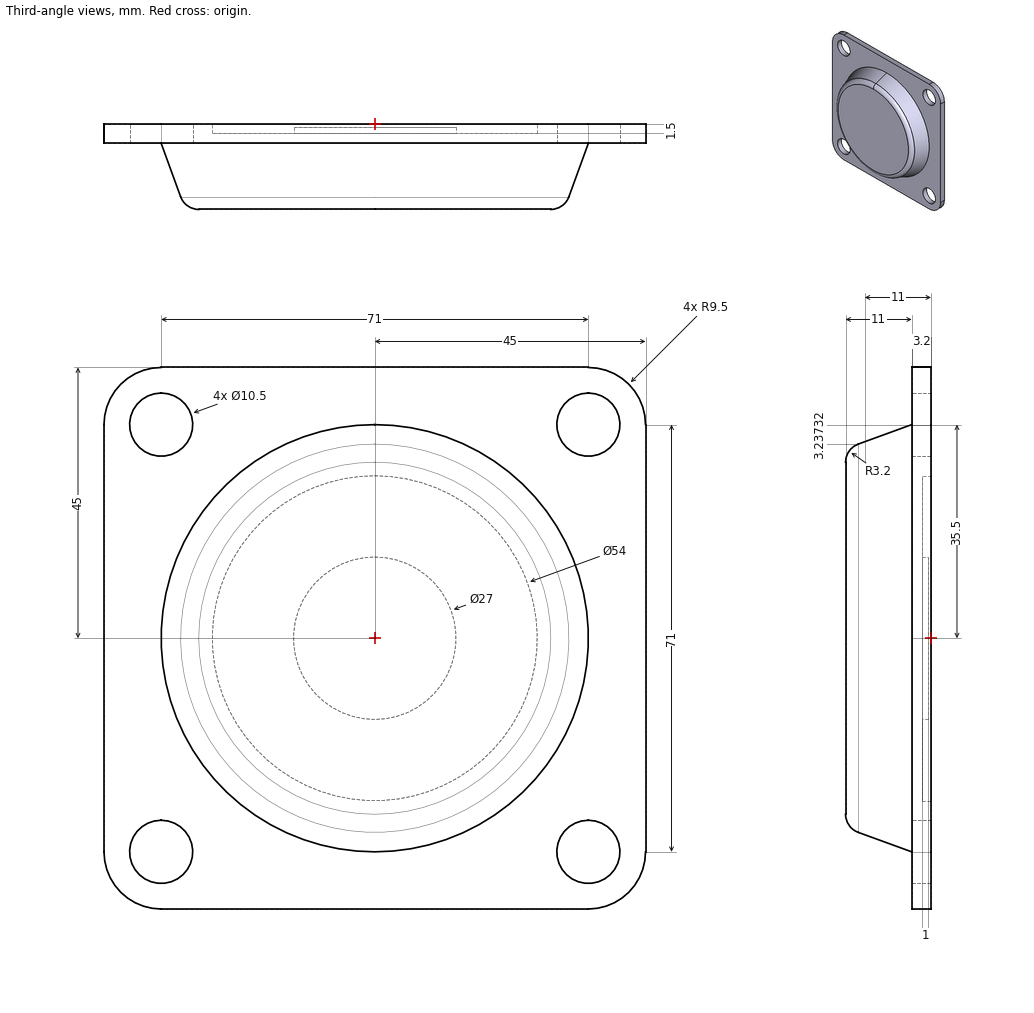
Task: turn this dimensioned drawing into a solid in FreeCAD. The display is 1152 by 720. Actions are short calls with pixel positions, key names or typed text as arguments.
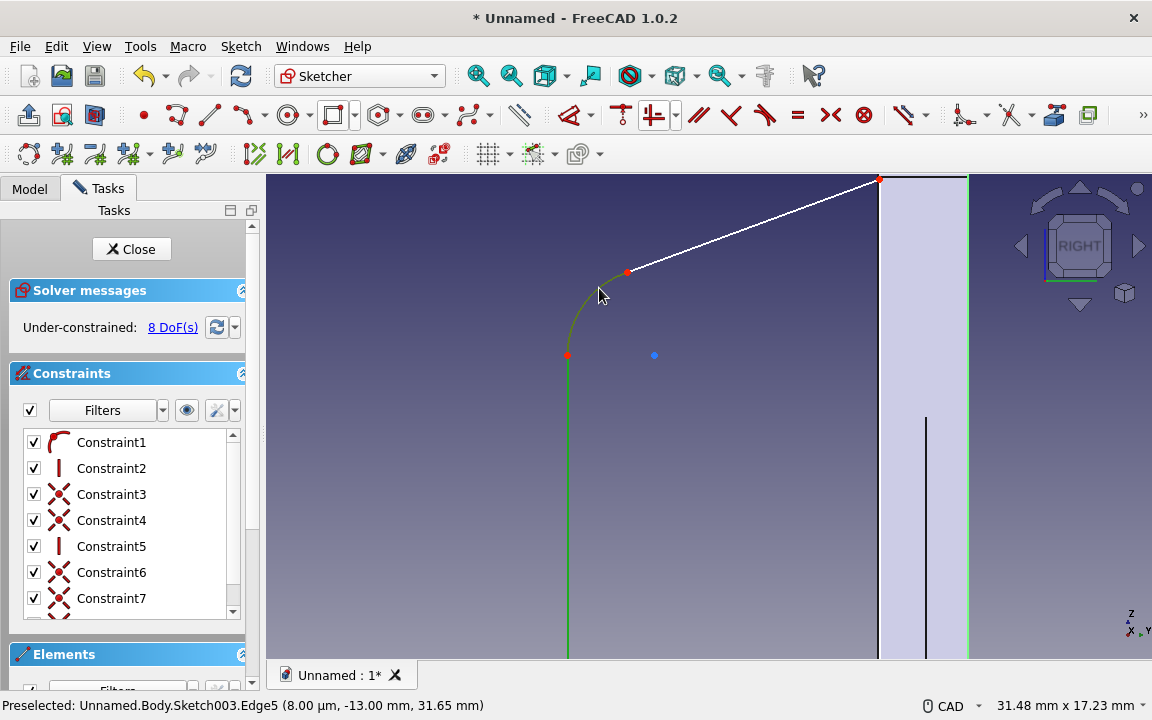
click(765, 116)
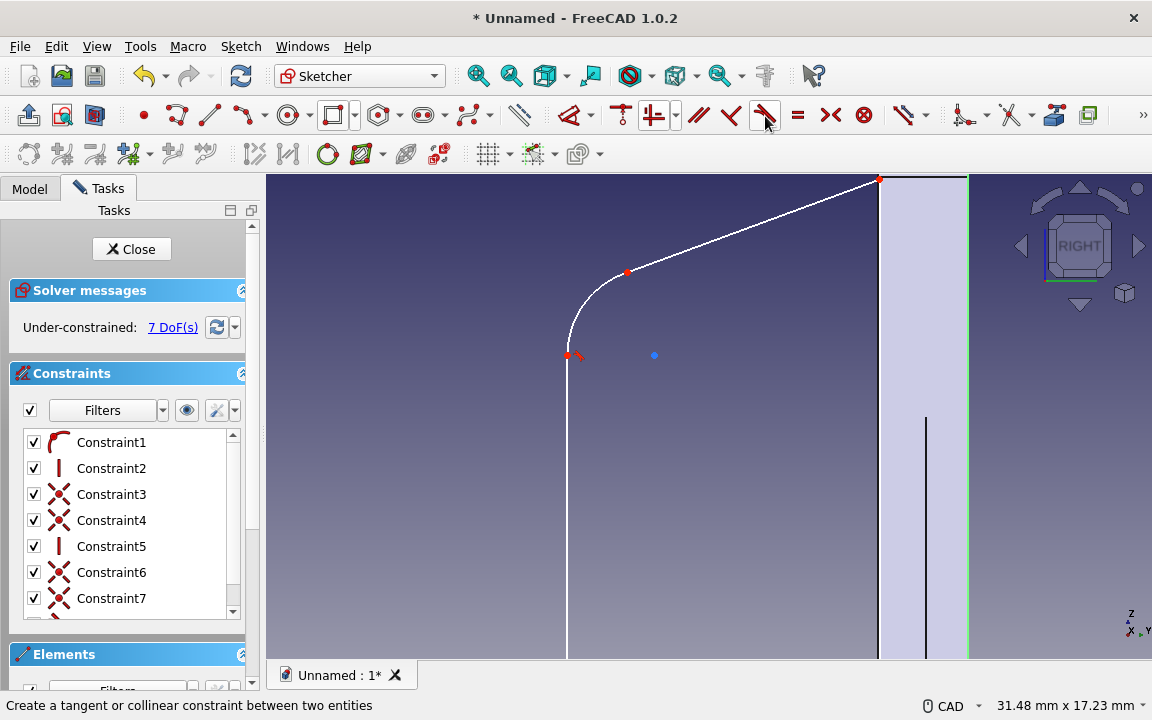
click(804, 207)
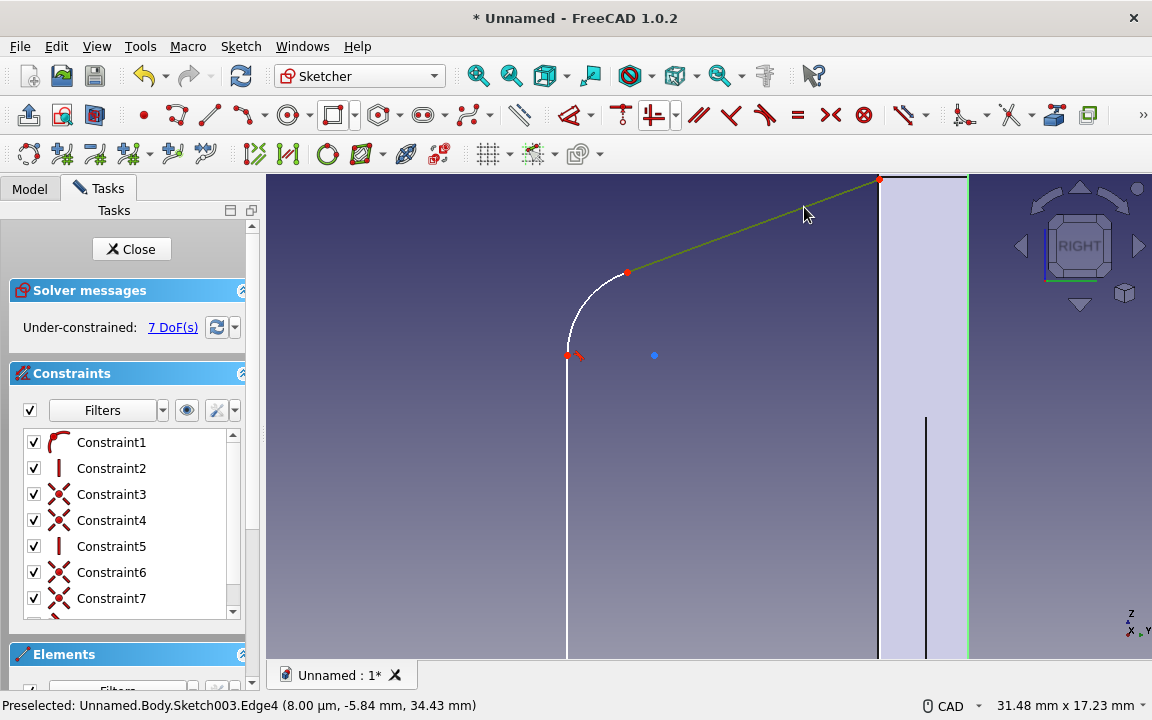
click(599, 288)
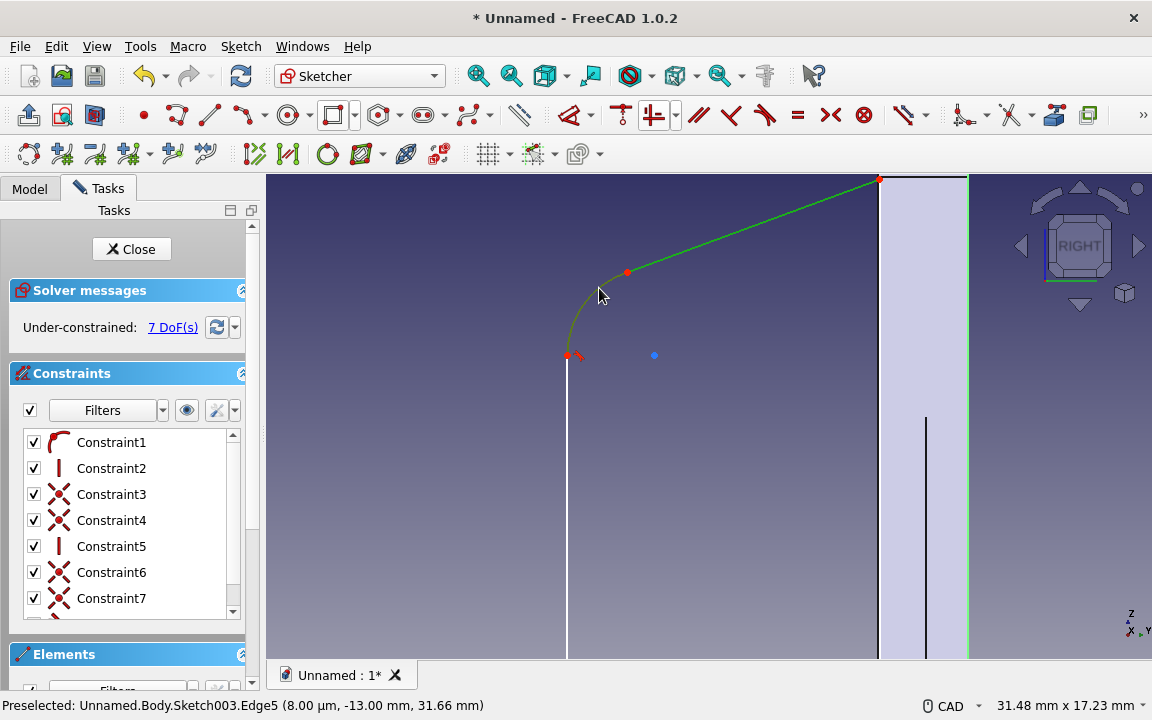
key(t)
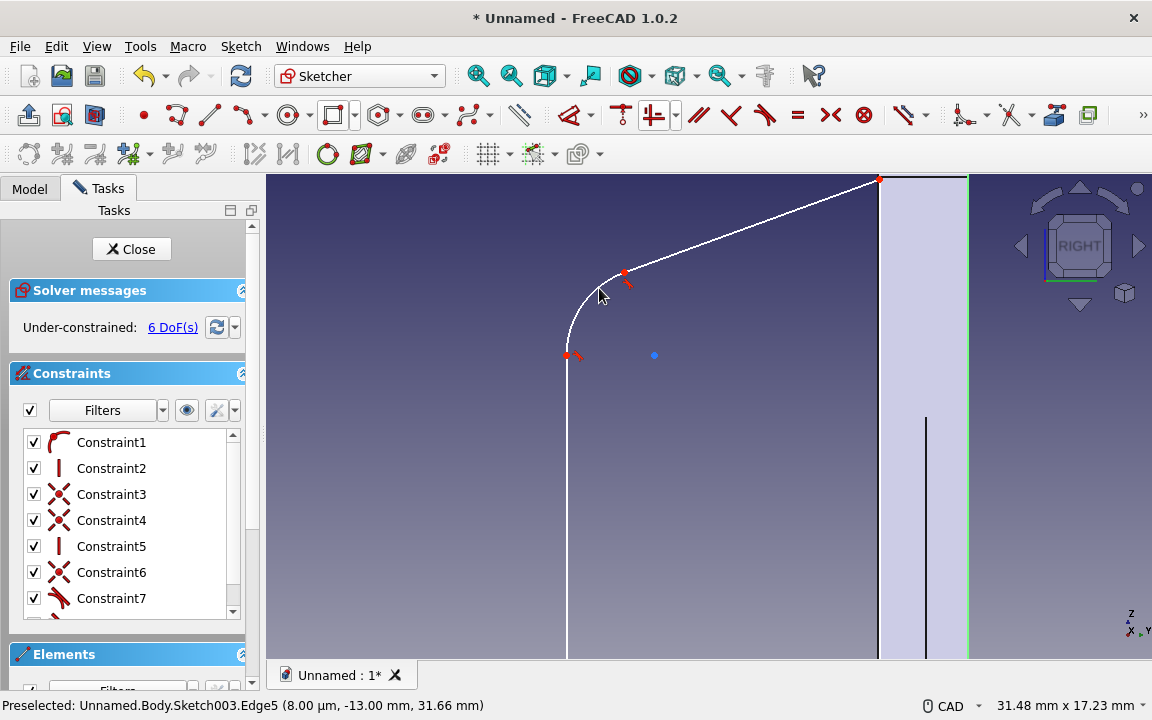
scroll(585, 304, down, 6)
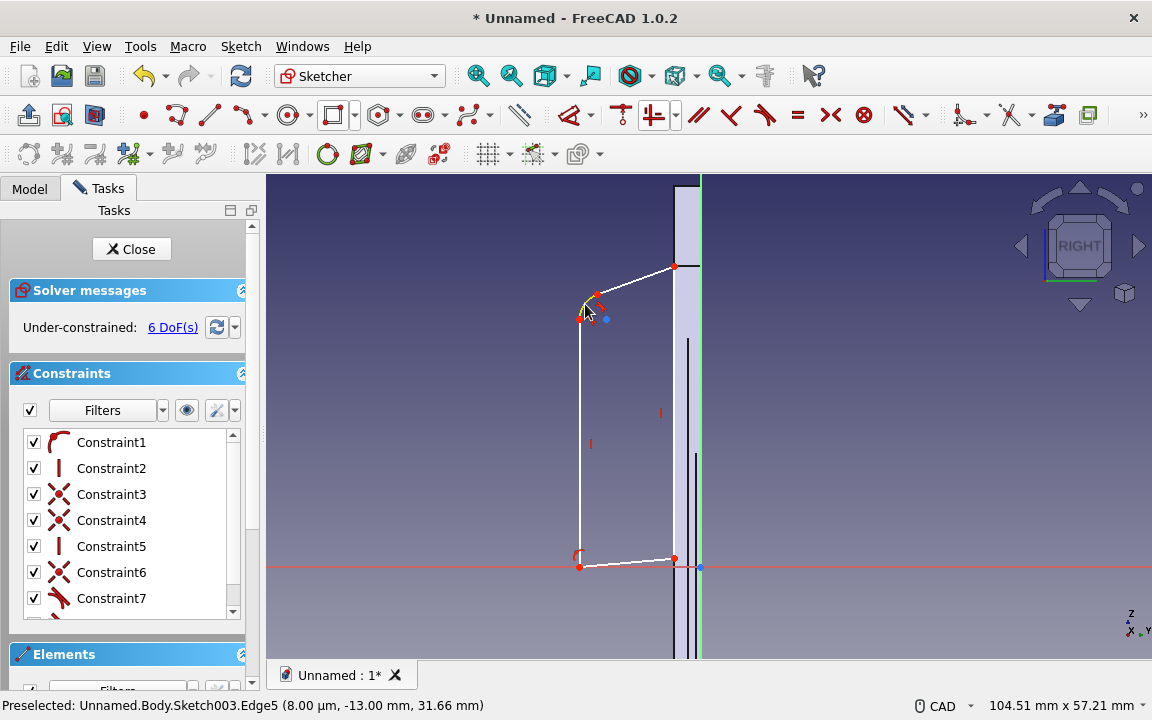
scroll(646, 561, up, 5)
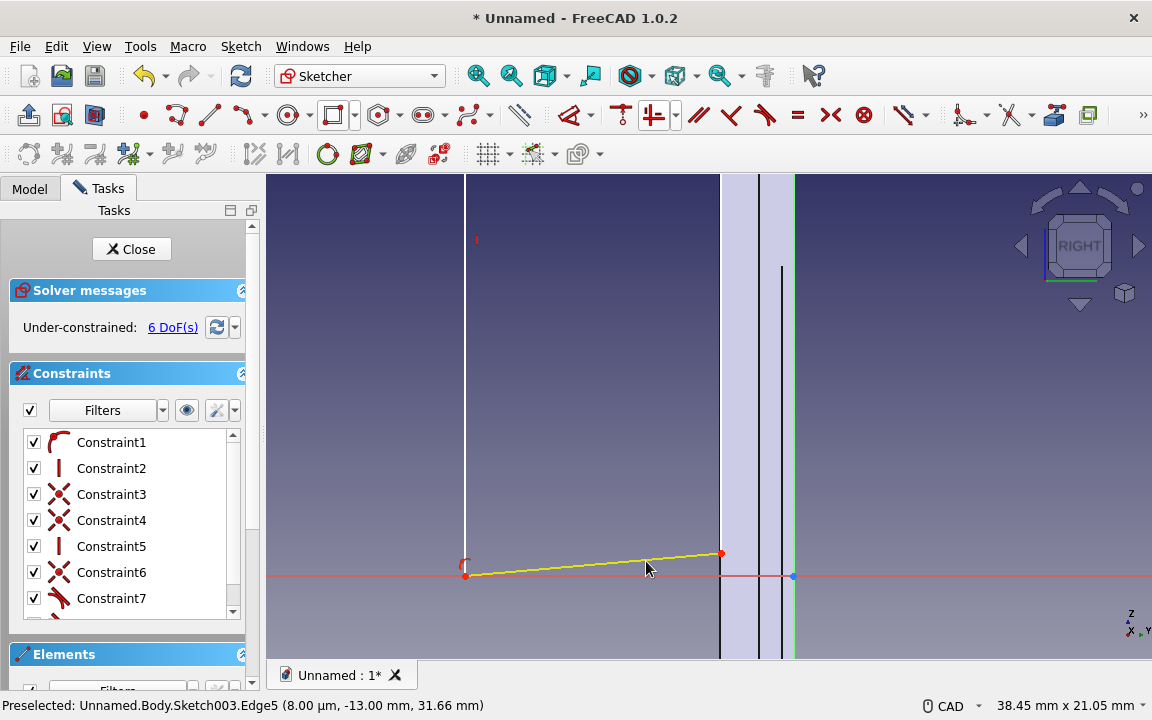
click(644, 560)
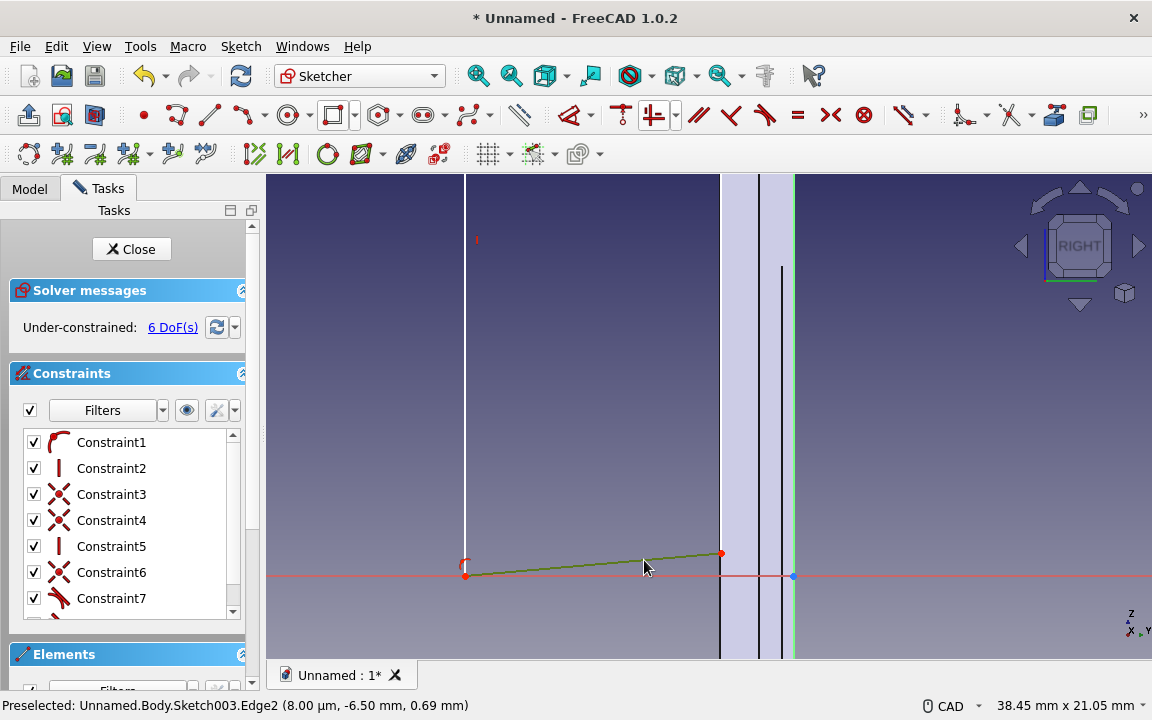
key(h)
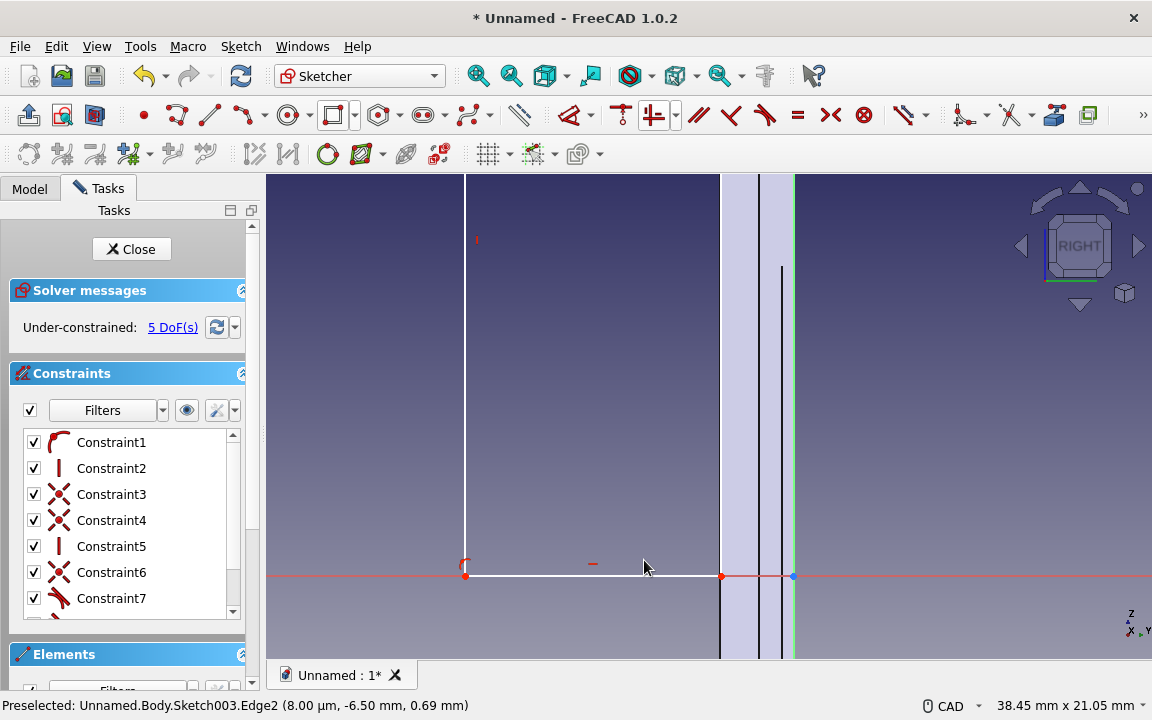
click(568, 116)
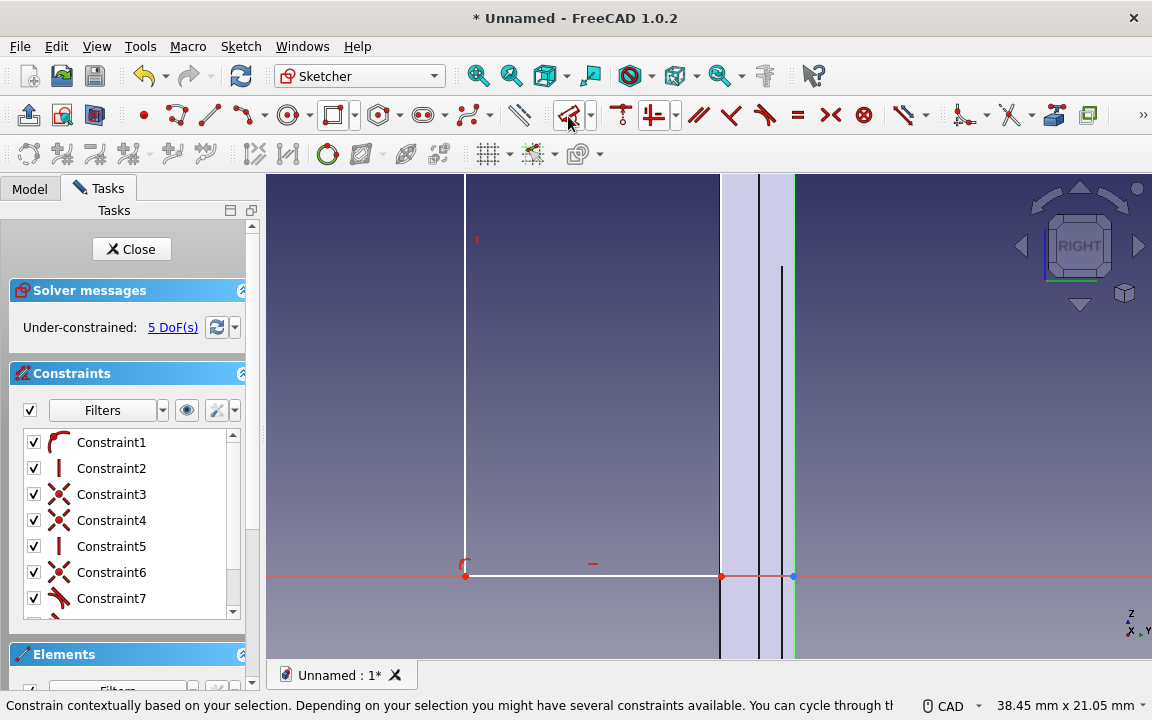
scroll(647, 562, down, 5)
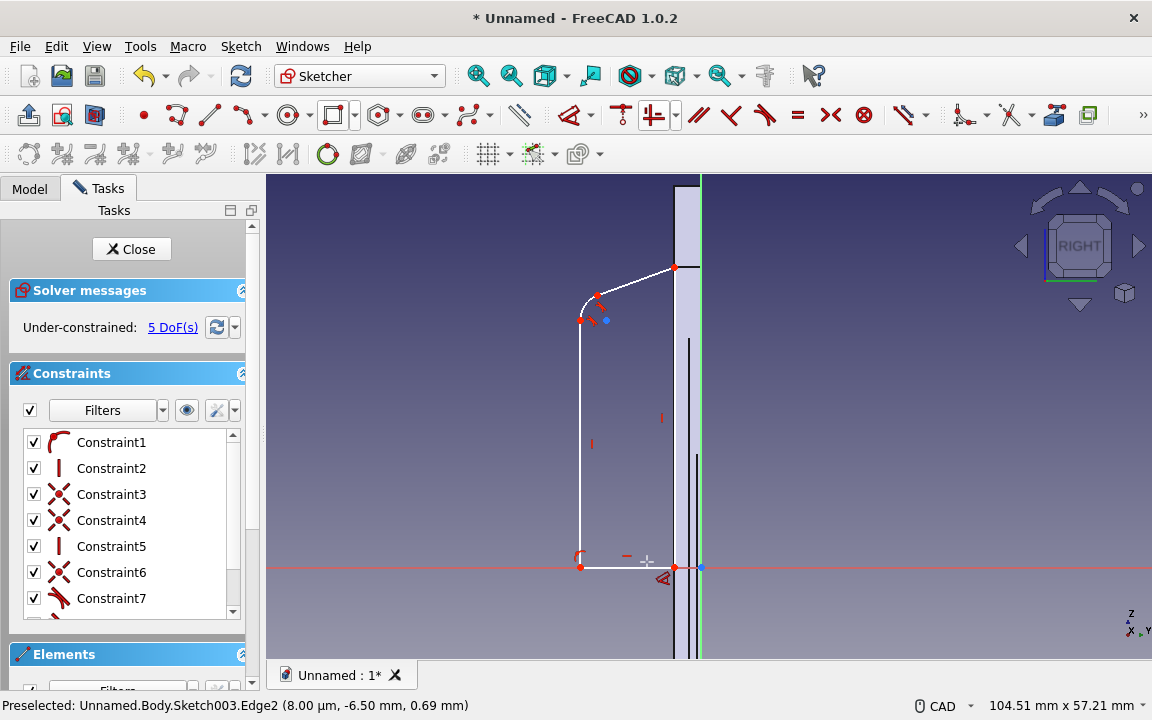
scroll(589, 300, up, 2)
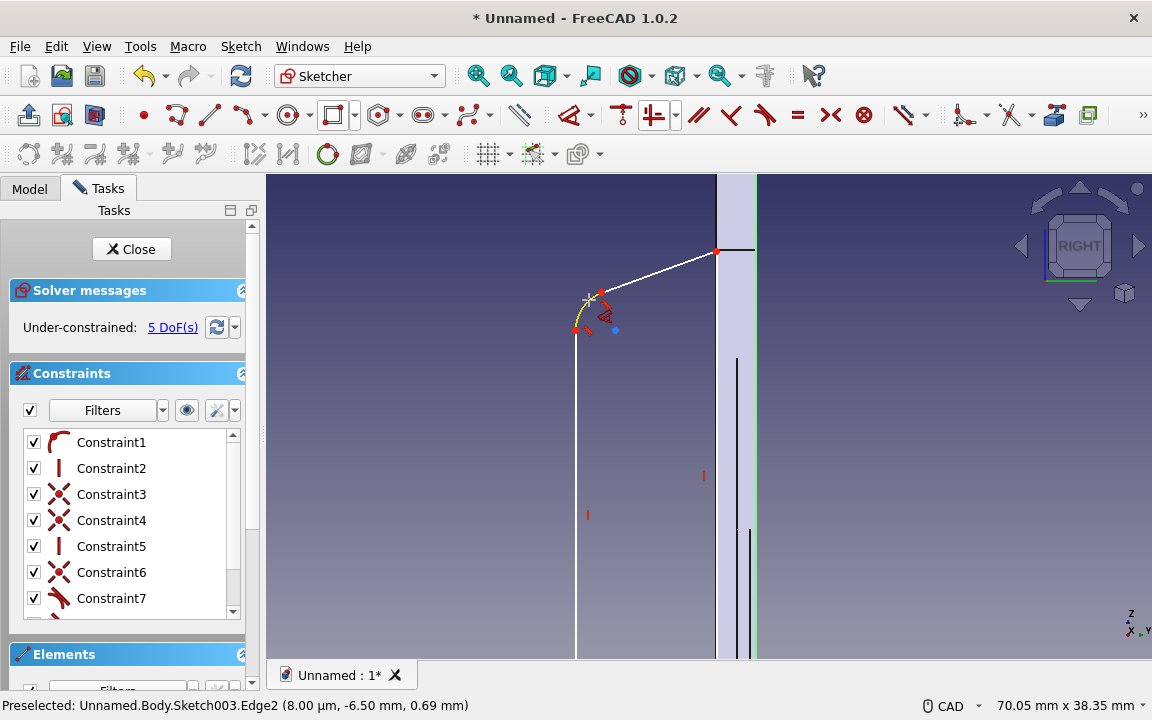
click(590, 300)
click(569, 276)